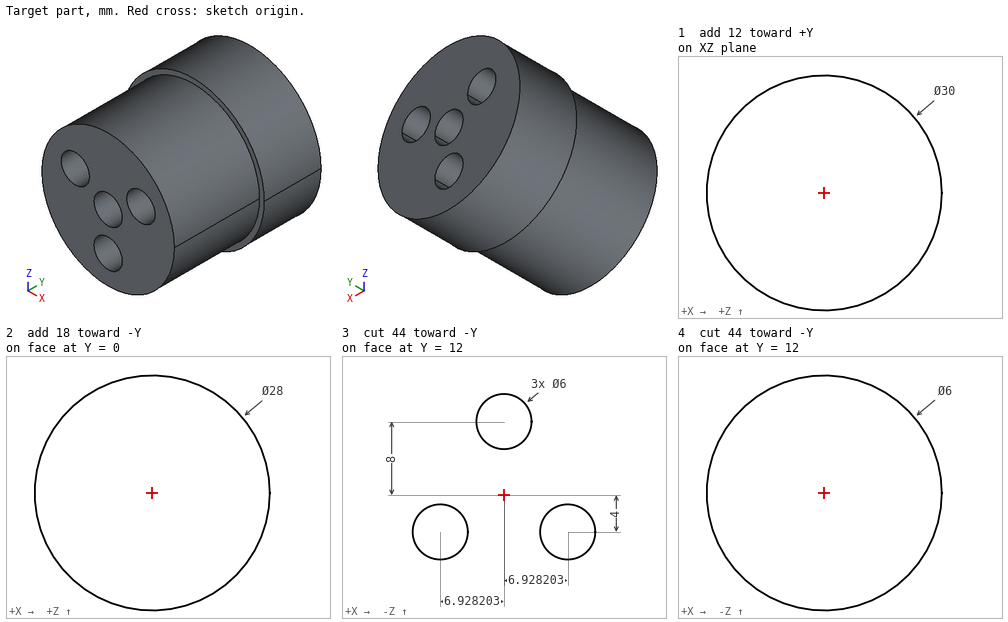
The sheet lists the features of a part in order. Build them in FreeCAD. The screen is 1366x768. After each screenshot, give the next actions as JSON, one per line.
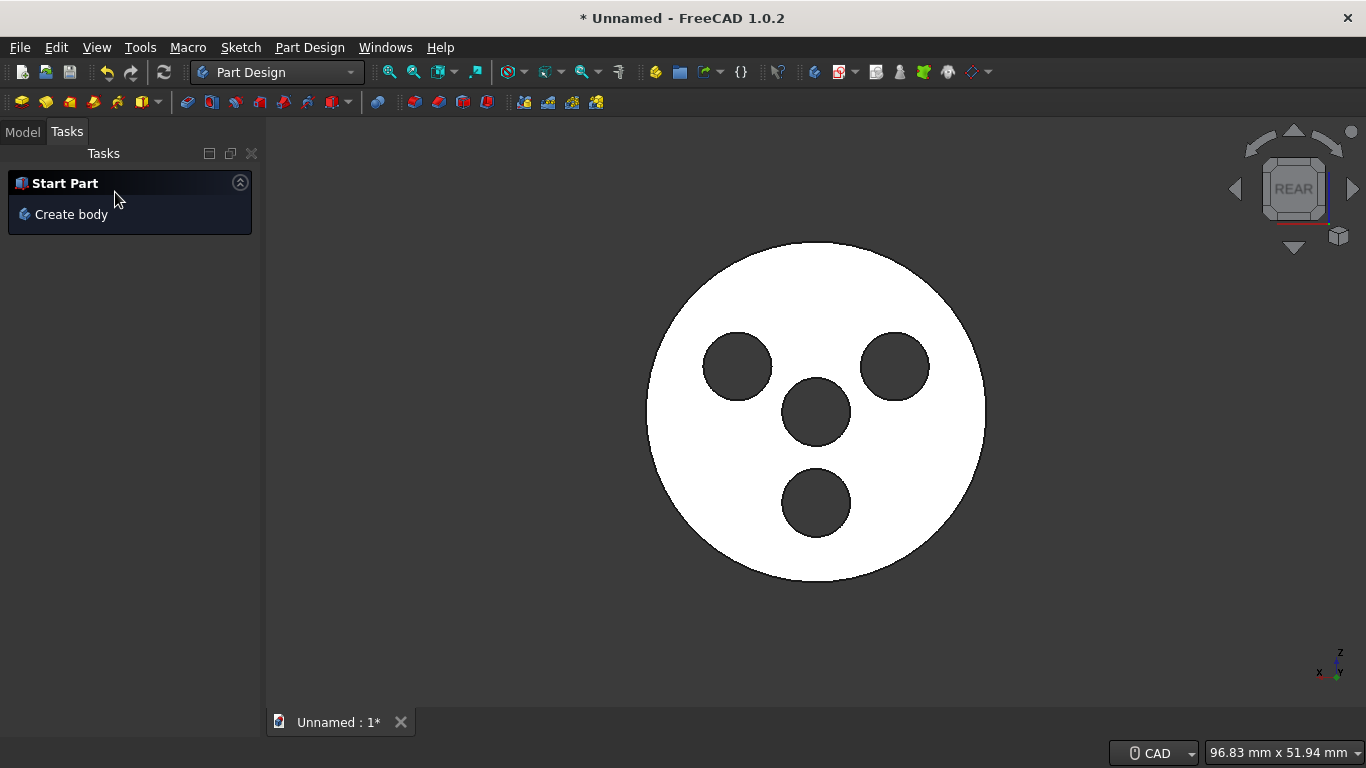
{"action": "key", "text": "0"}